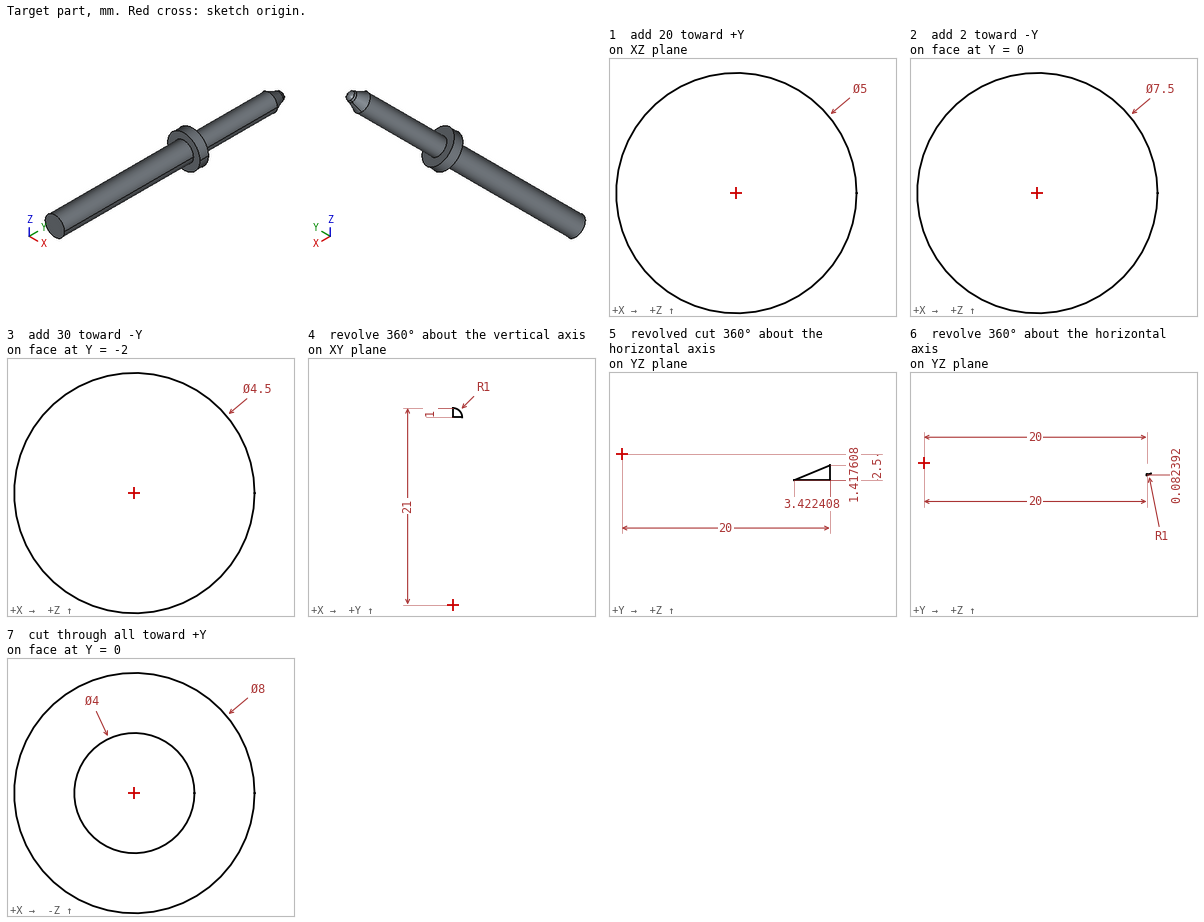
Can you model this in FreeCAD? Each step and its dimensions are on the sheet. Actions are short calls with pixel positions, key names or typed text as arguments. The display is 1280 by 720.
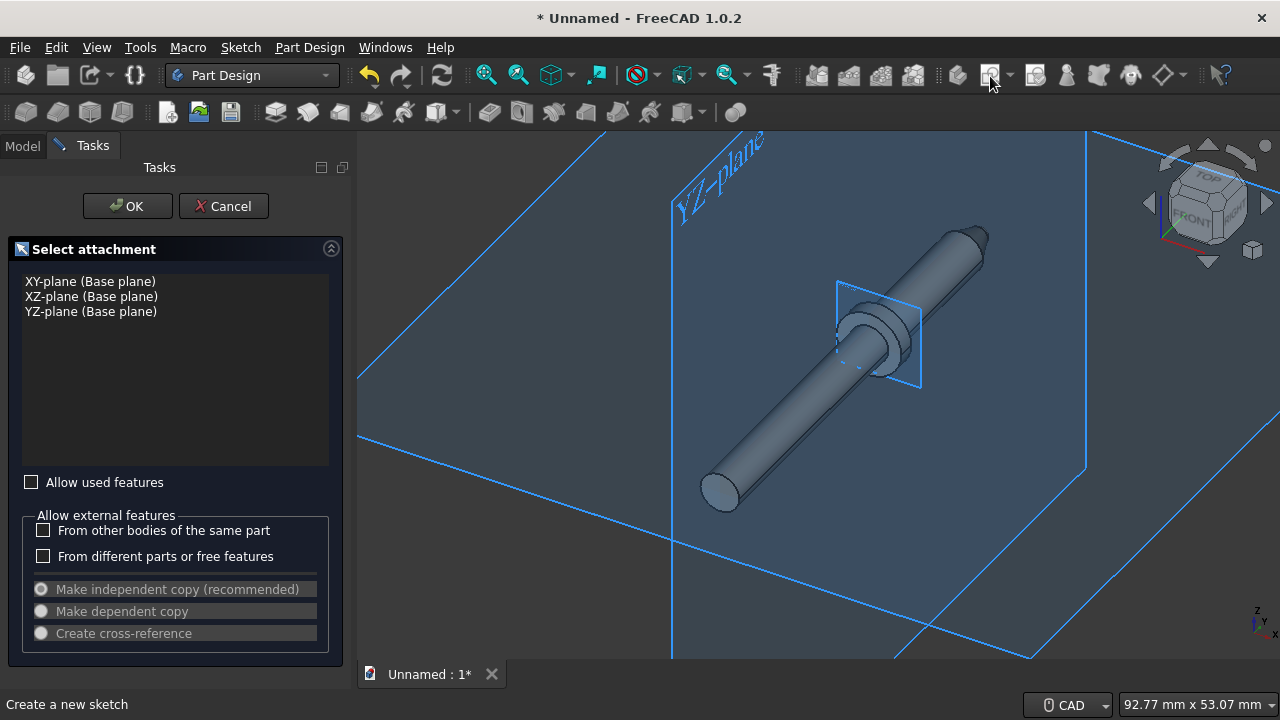
click(82, 312)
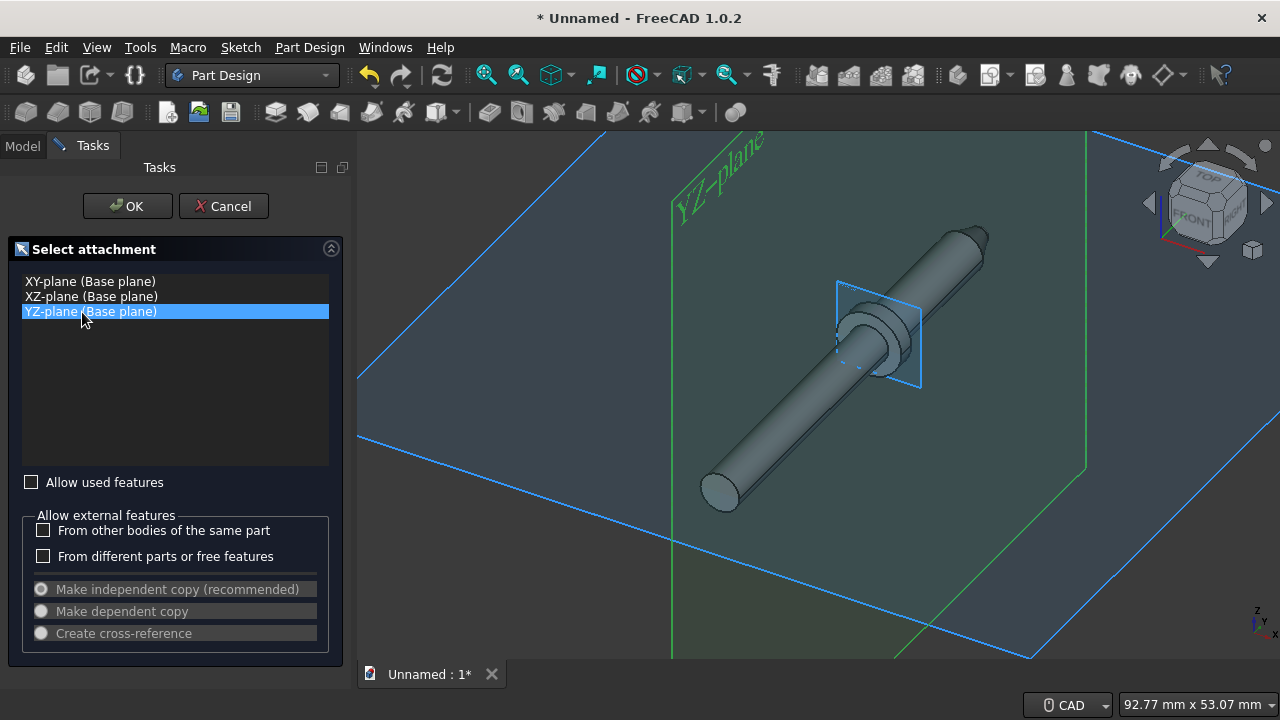
click(128, 206)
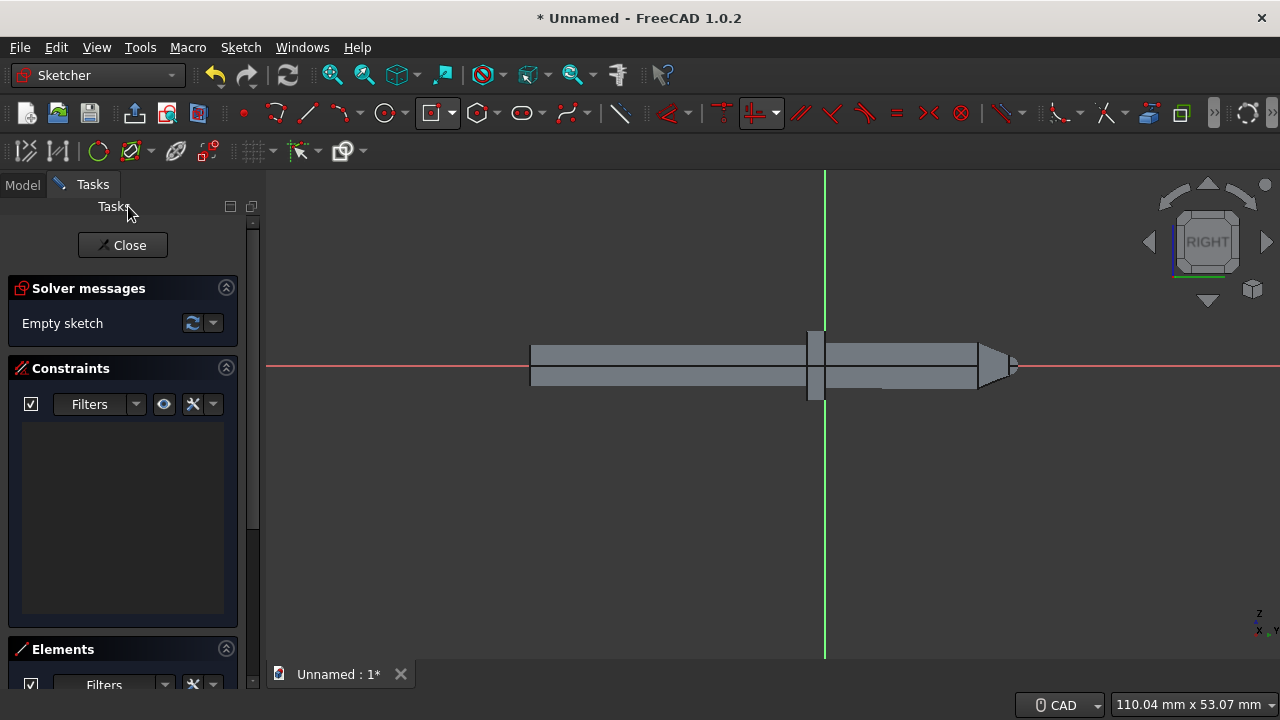
click(200, 114)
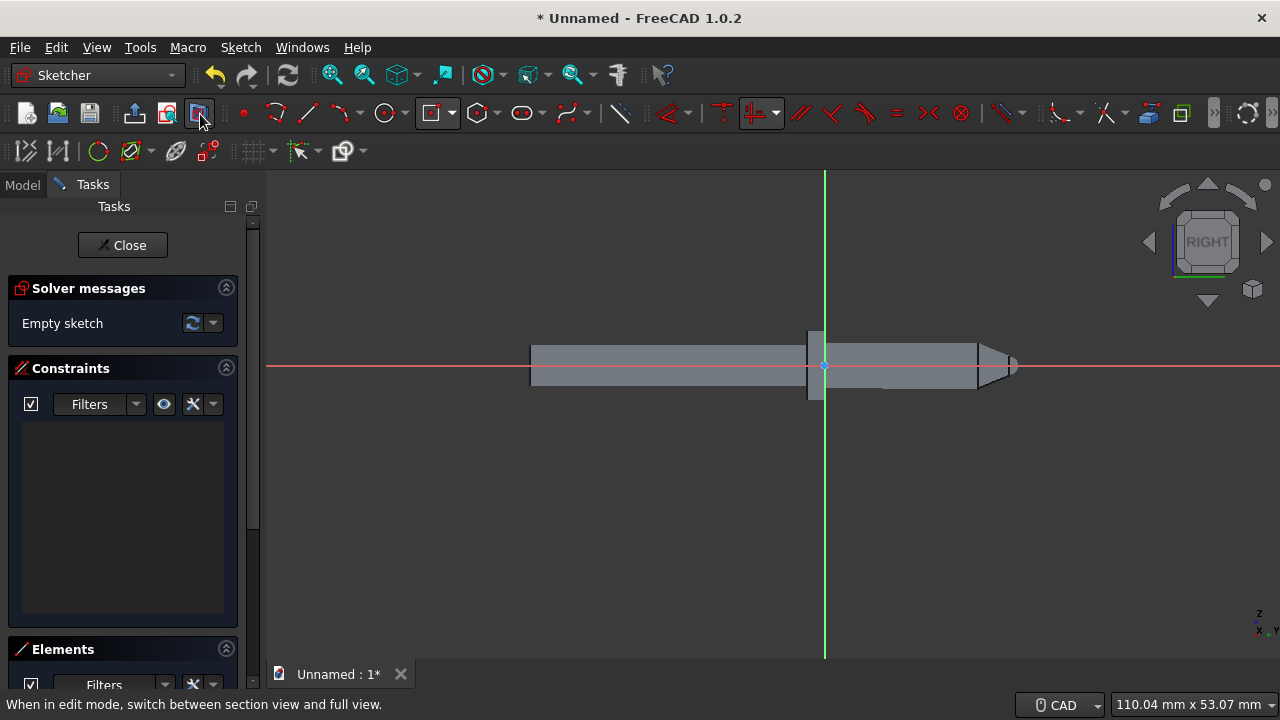
scroll(1027, 373, up, 15)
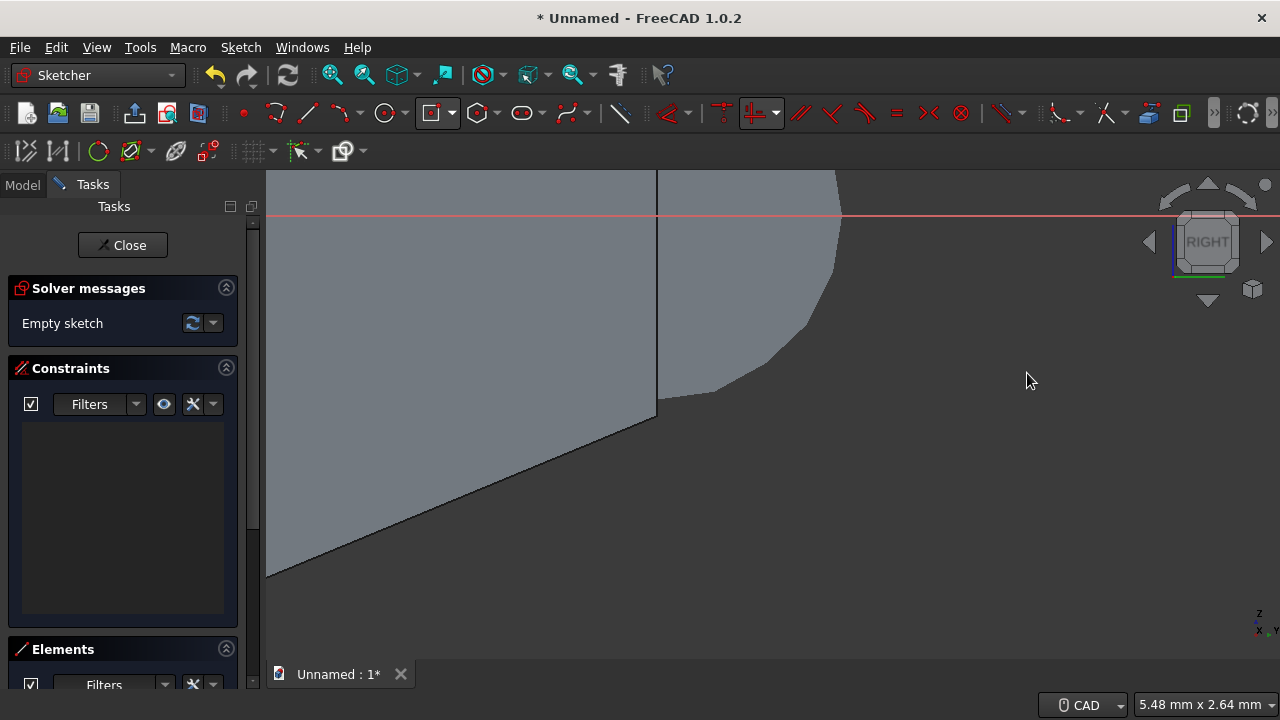
scroll(691, 400, up, 11)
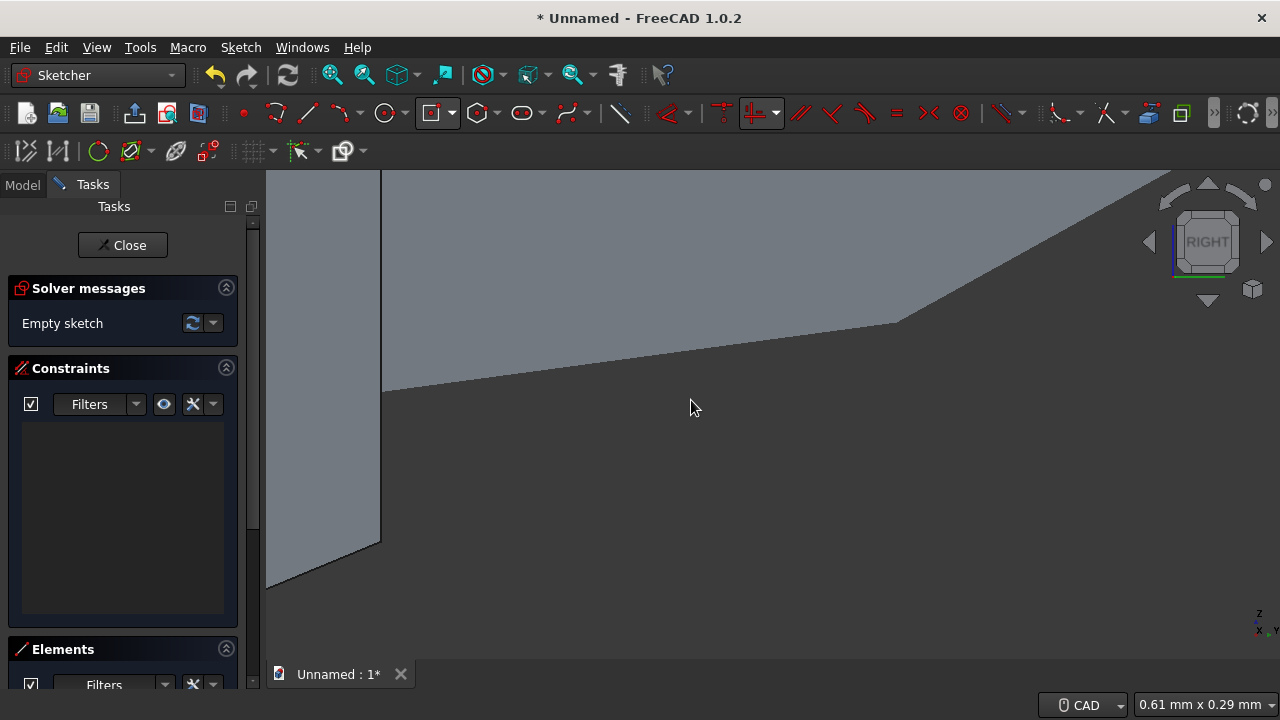
click(276, 114)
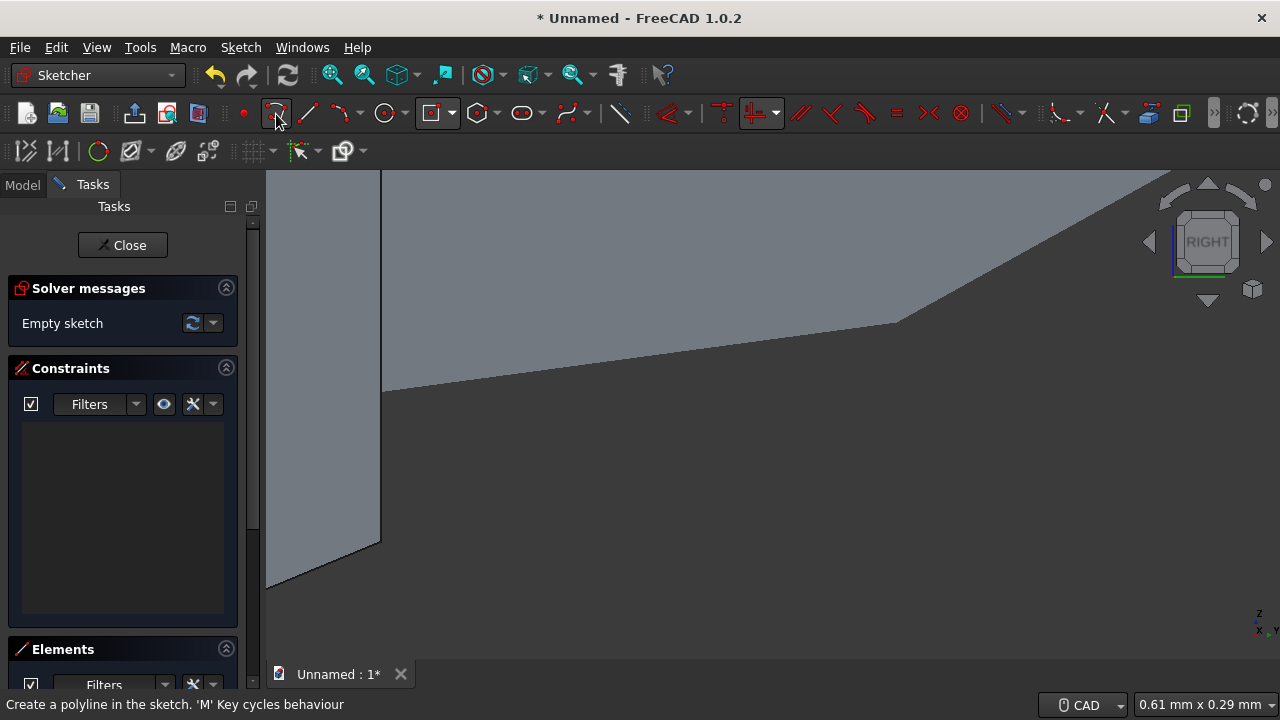
click(381, 404)
click(381, 542)
click(1020, 277)
right_click(1020, 277)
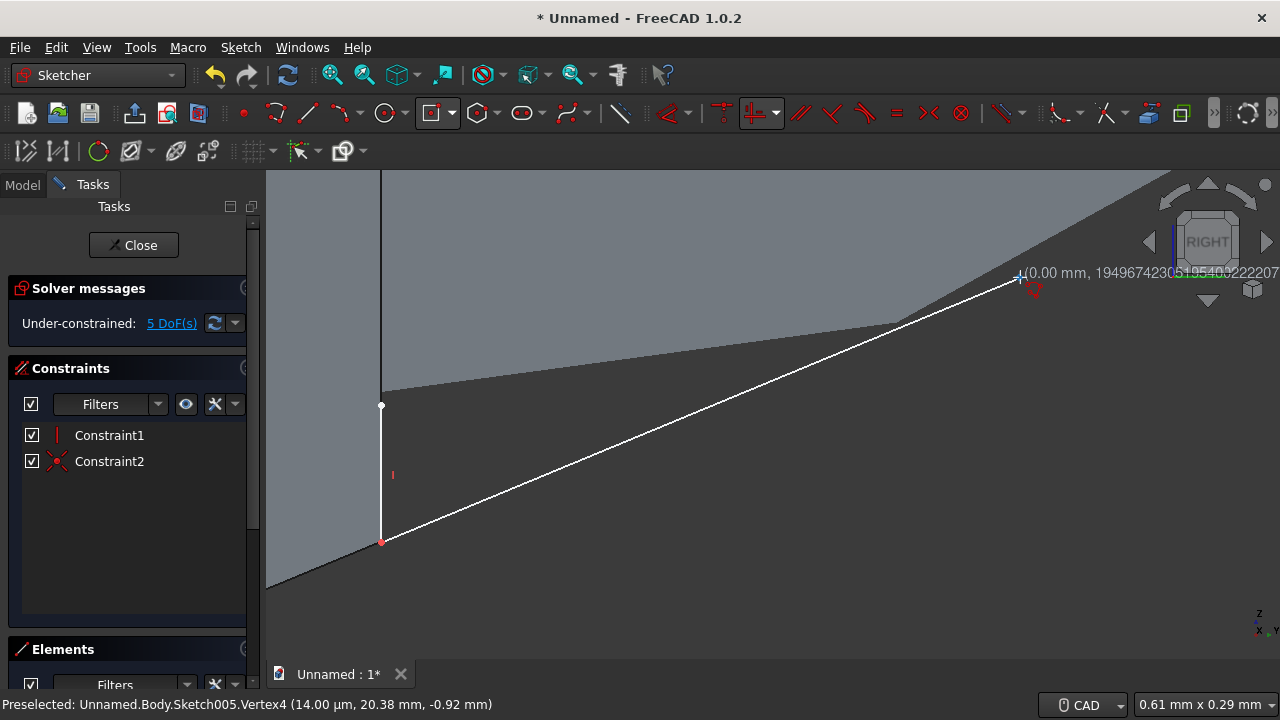
click(340, 114)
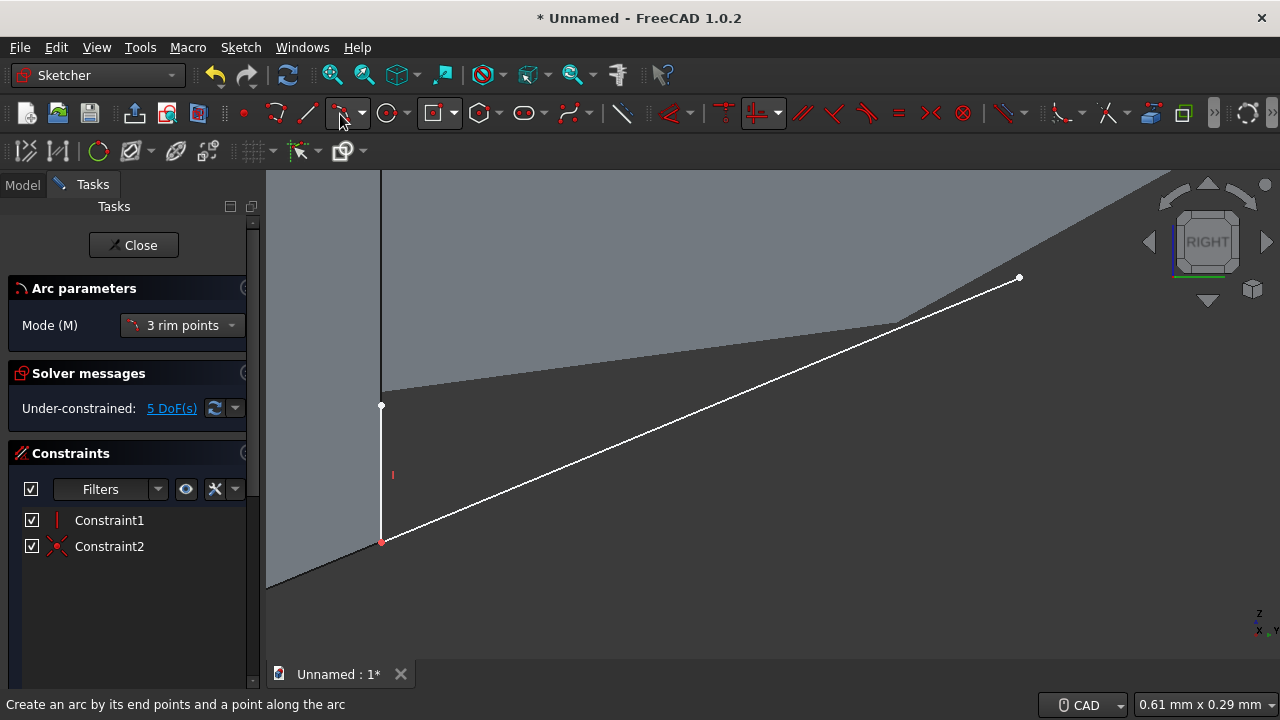
click(1020, 278)
click(381, 405)
click(707, 372)
key(Escape)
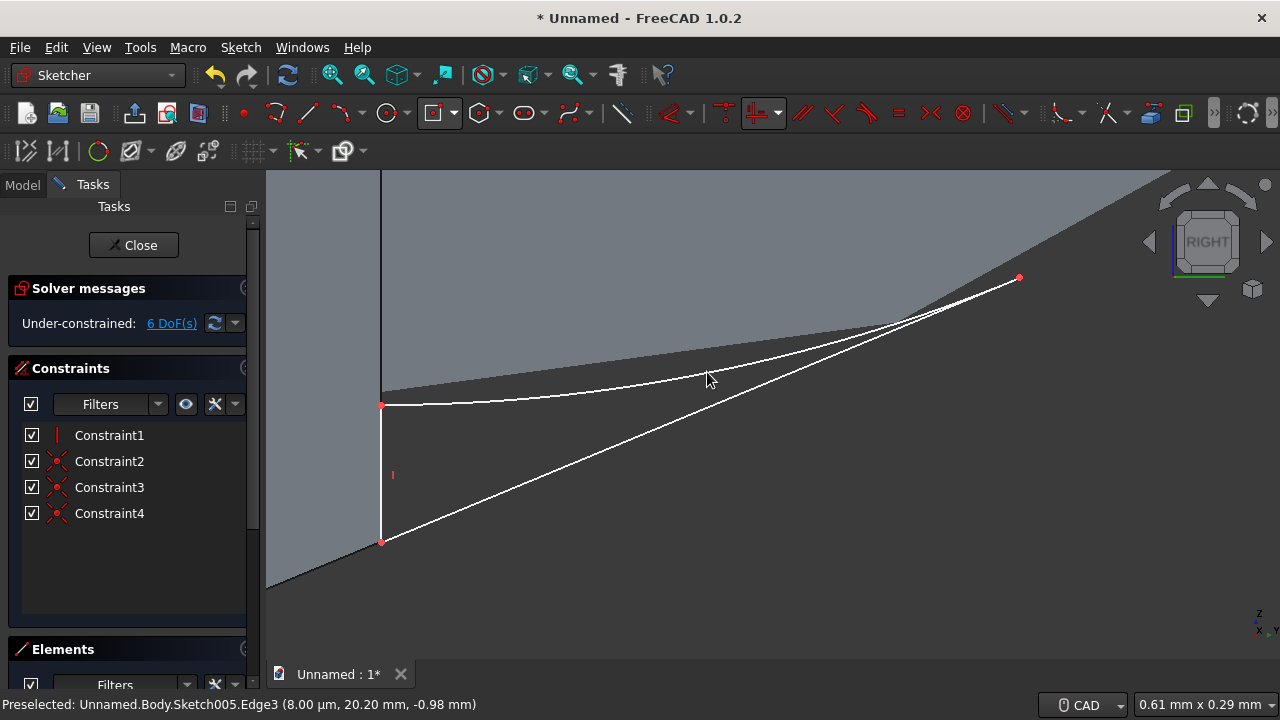
click(573, 463)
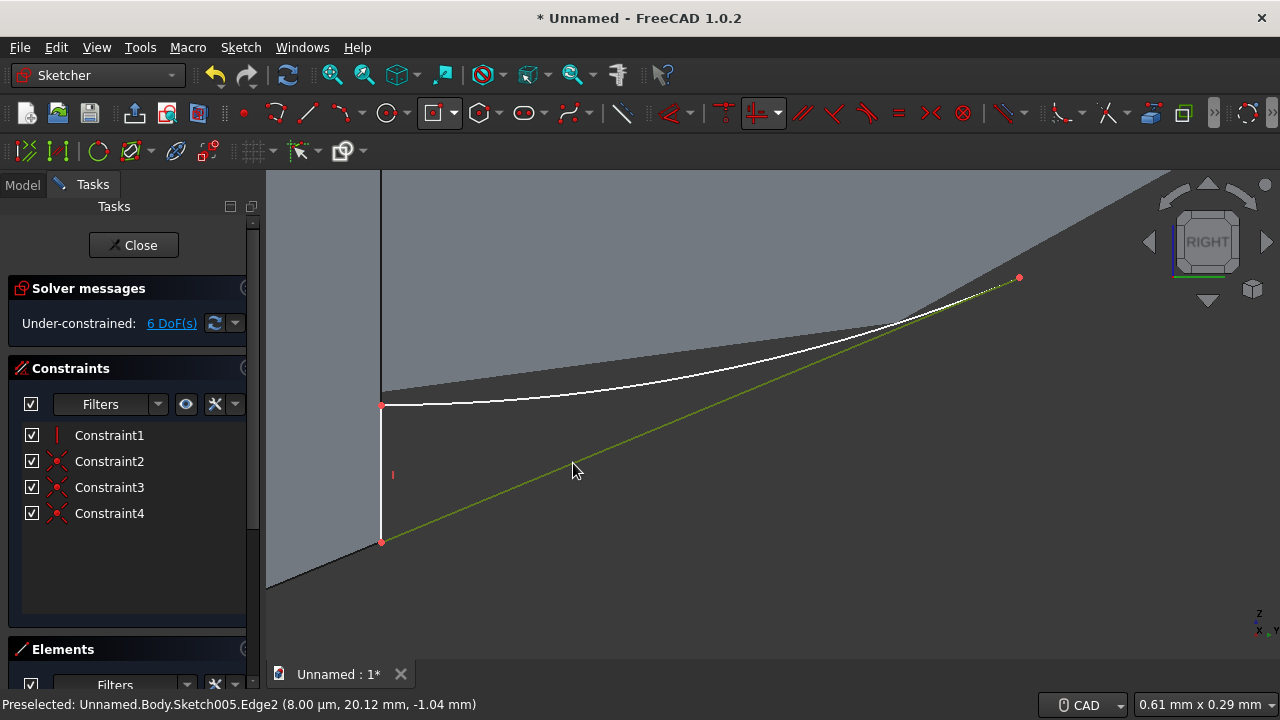
click(577, 394)